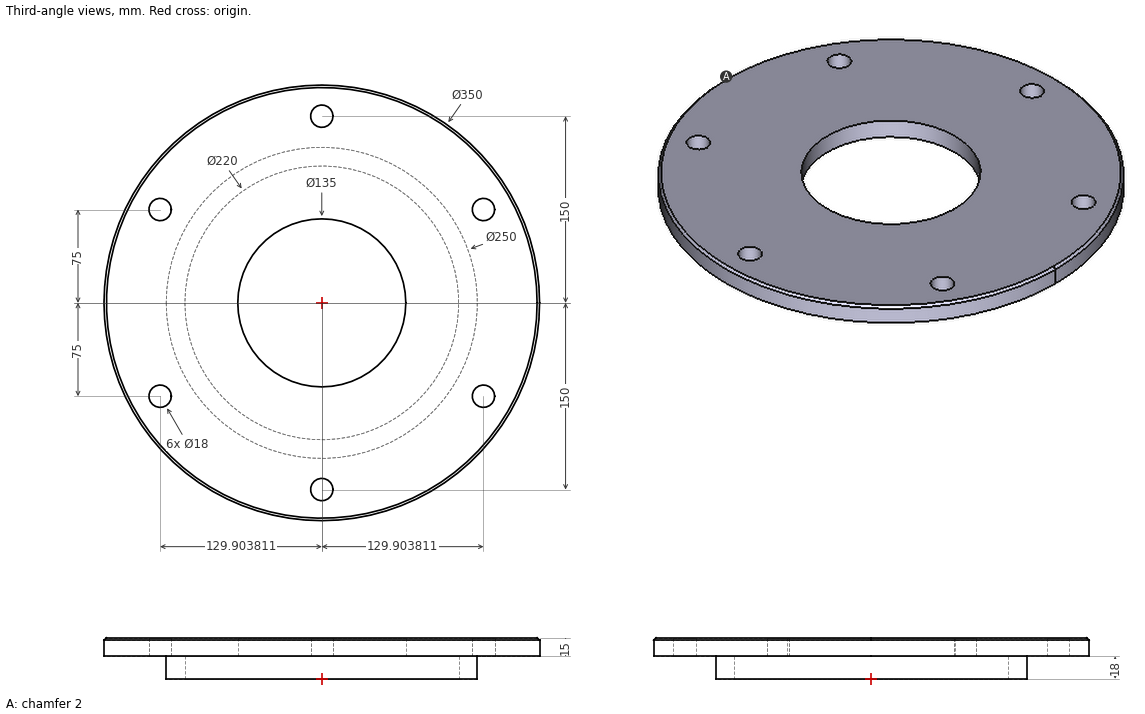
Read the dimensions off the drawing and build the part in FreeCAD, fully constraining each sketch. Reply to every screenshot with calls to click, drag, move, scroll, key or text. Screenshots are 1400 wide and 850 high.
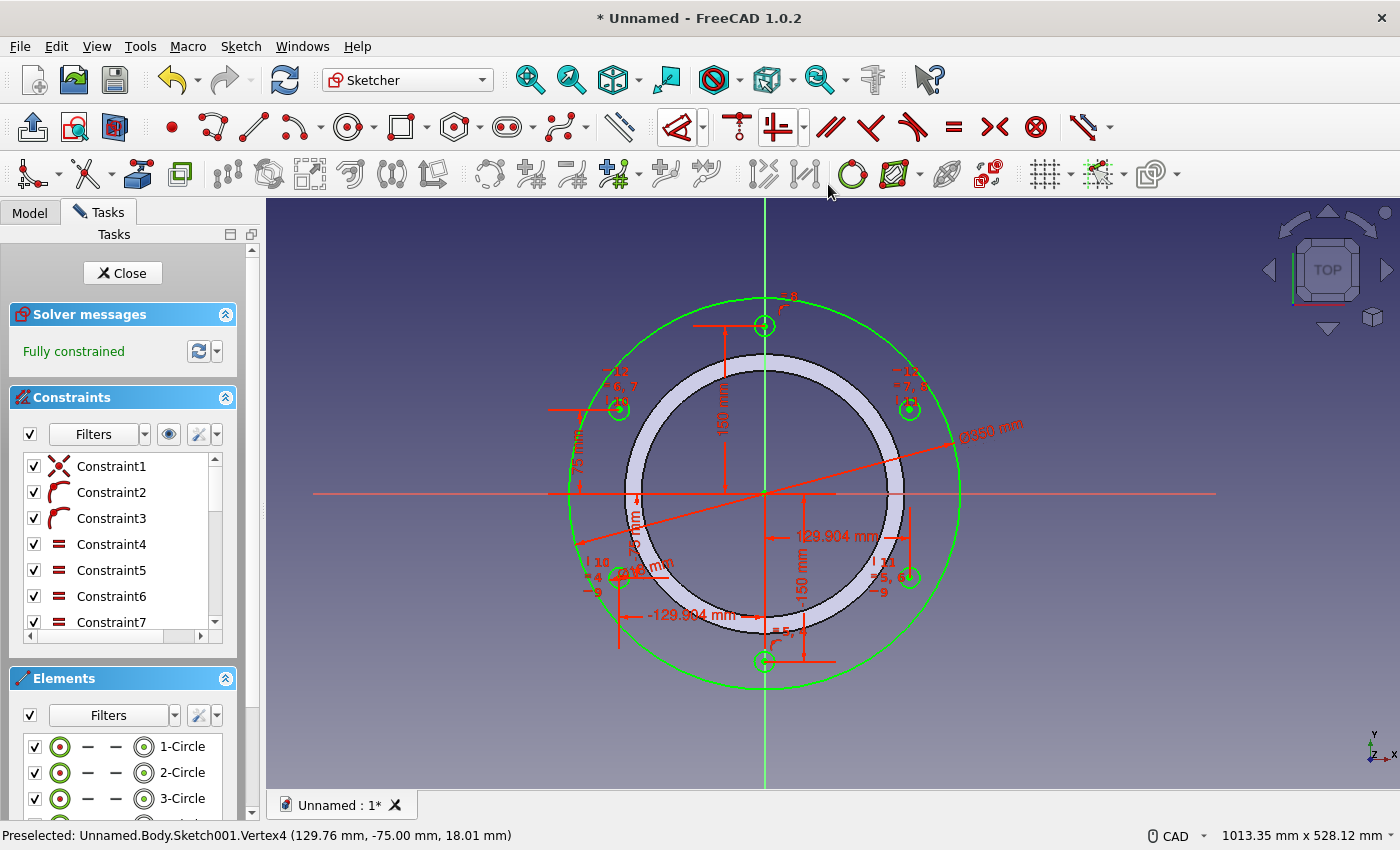
click(123, 273)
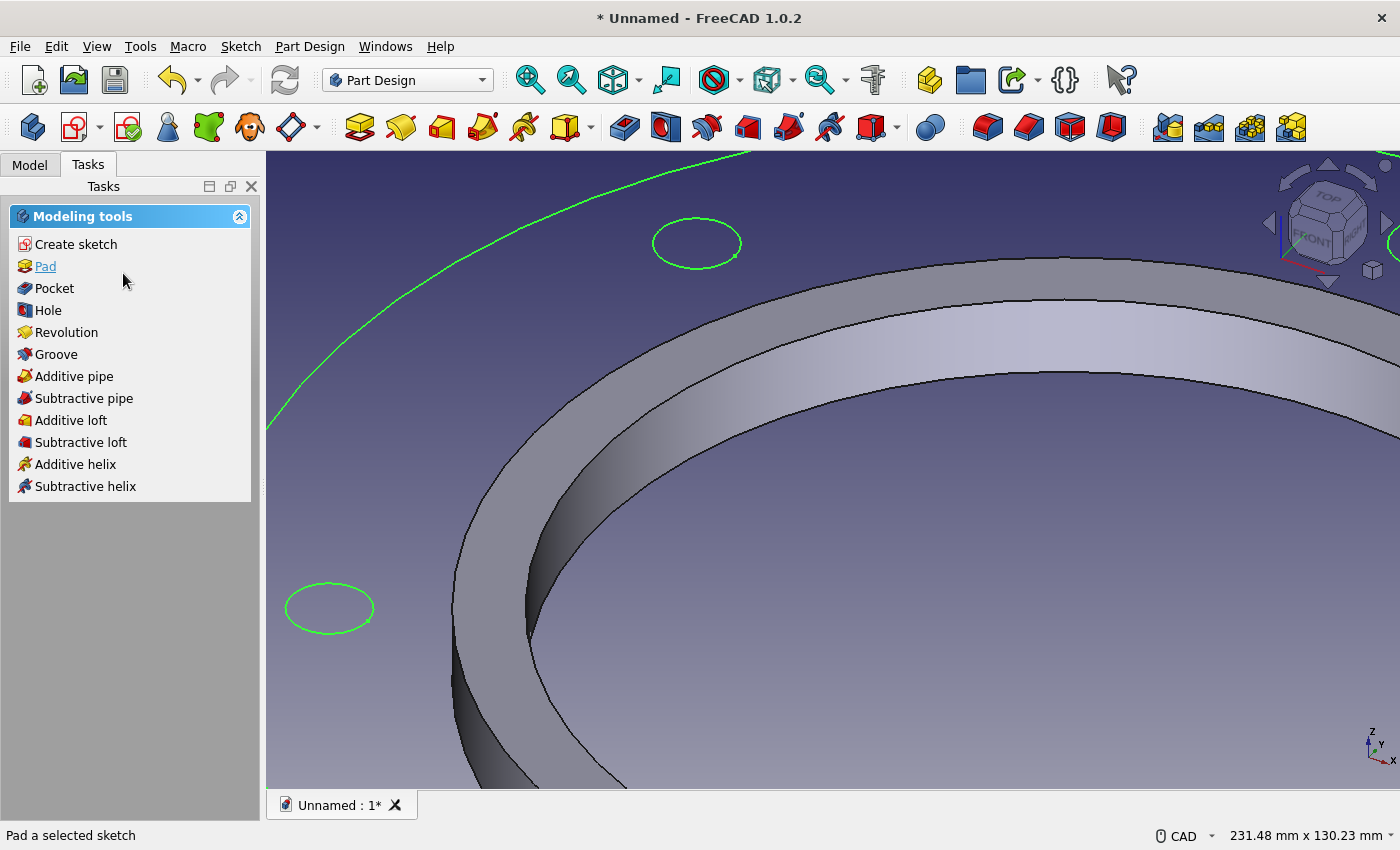
click(360, 128)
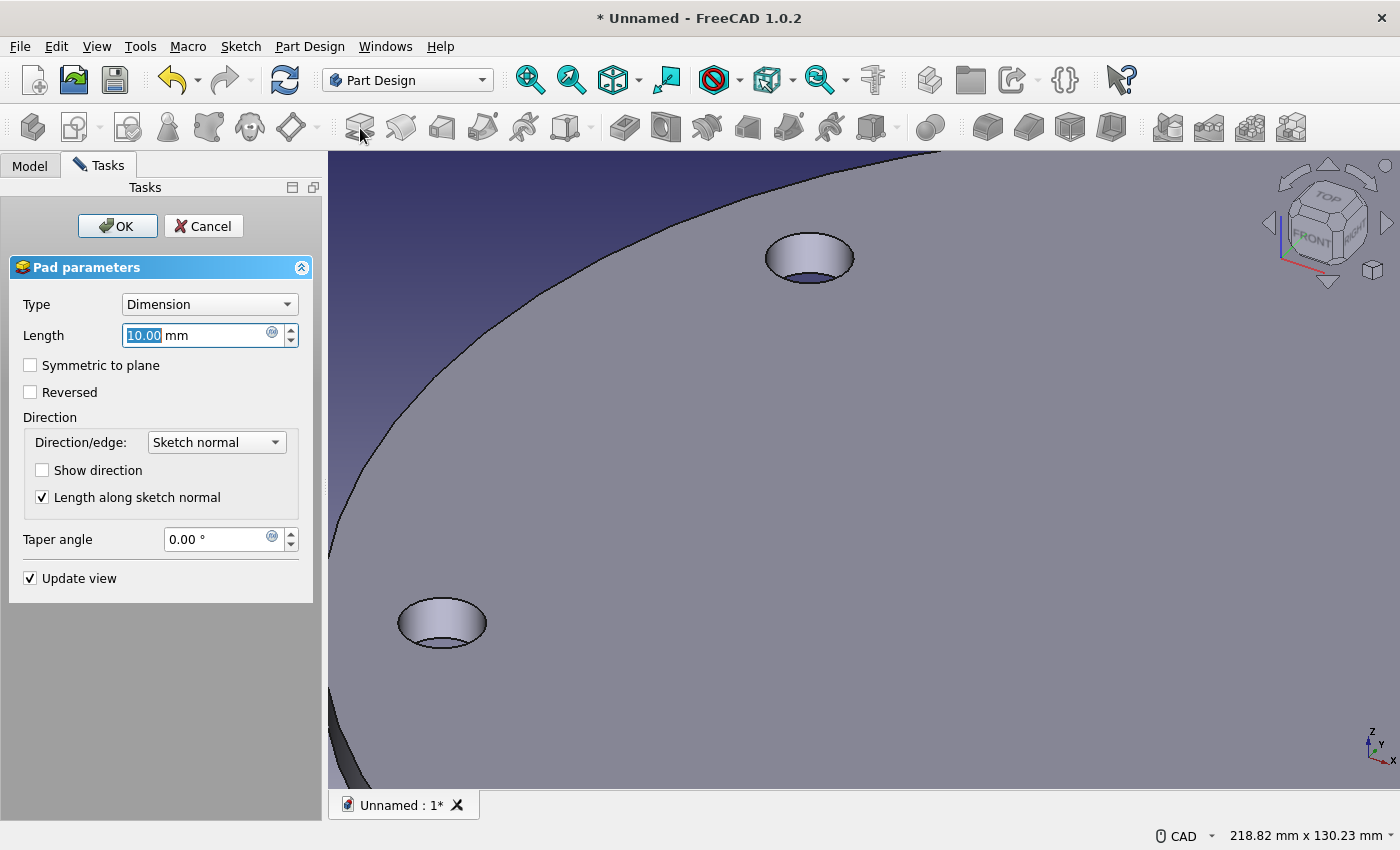
text(15)
key(Tab)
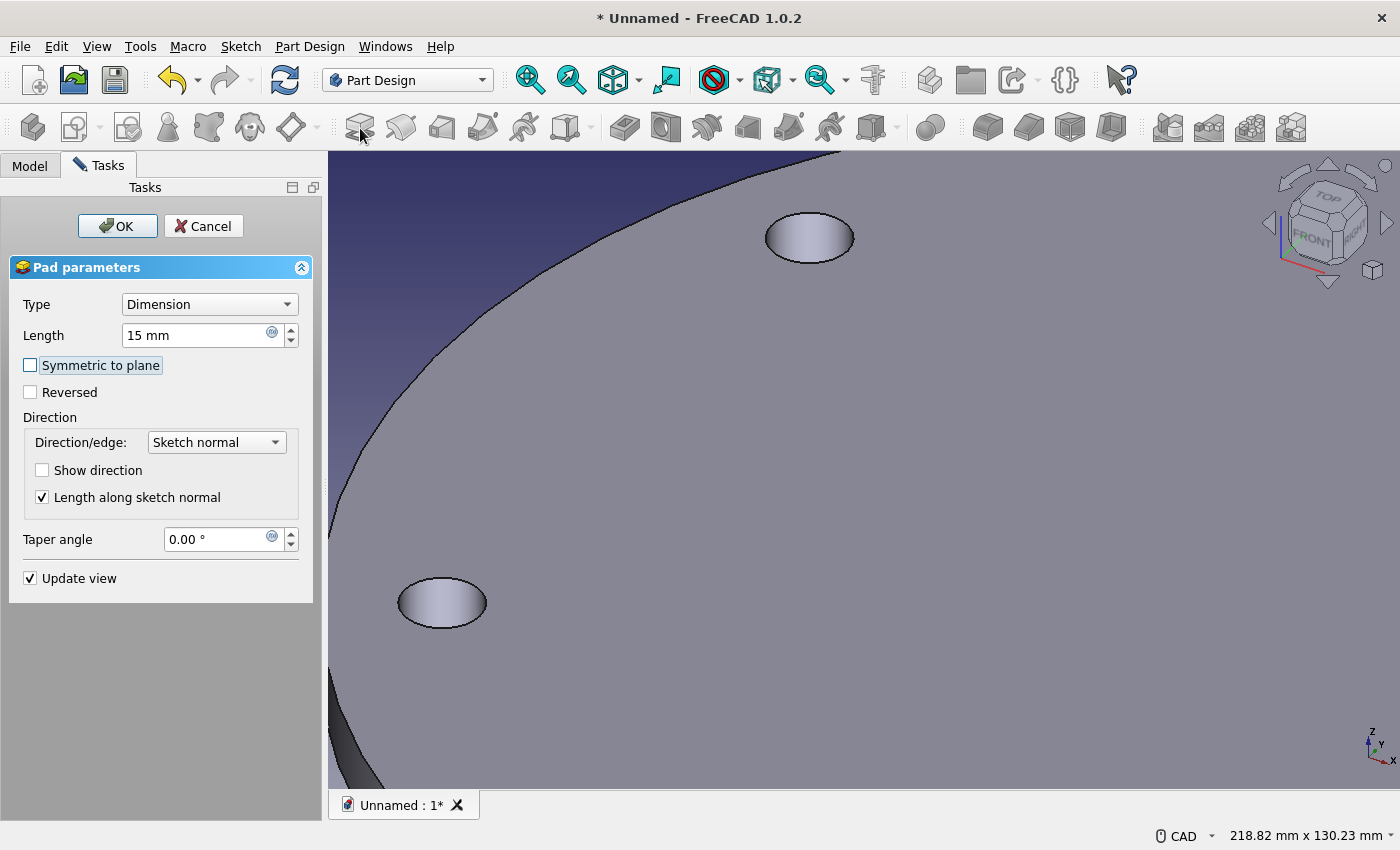
click(118, 226)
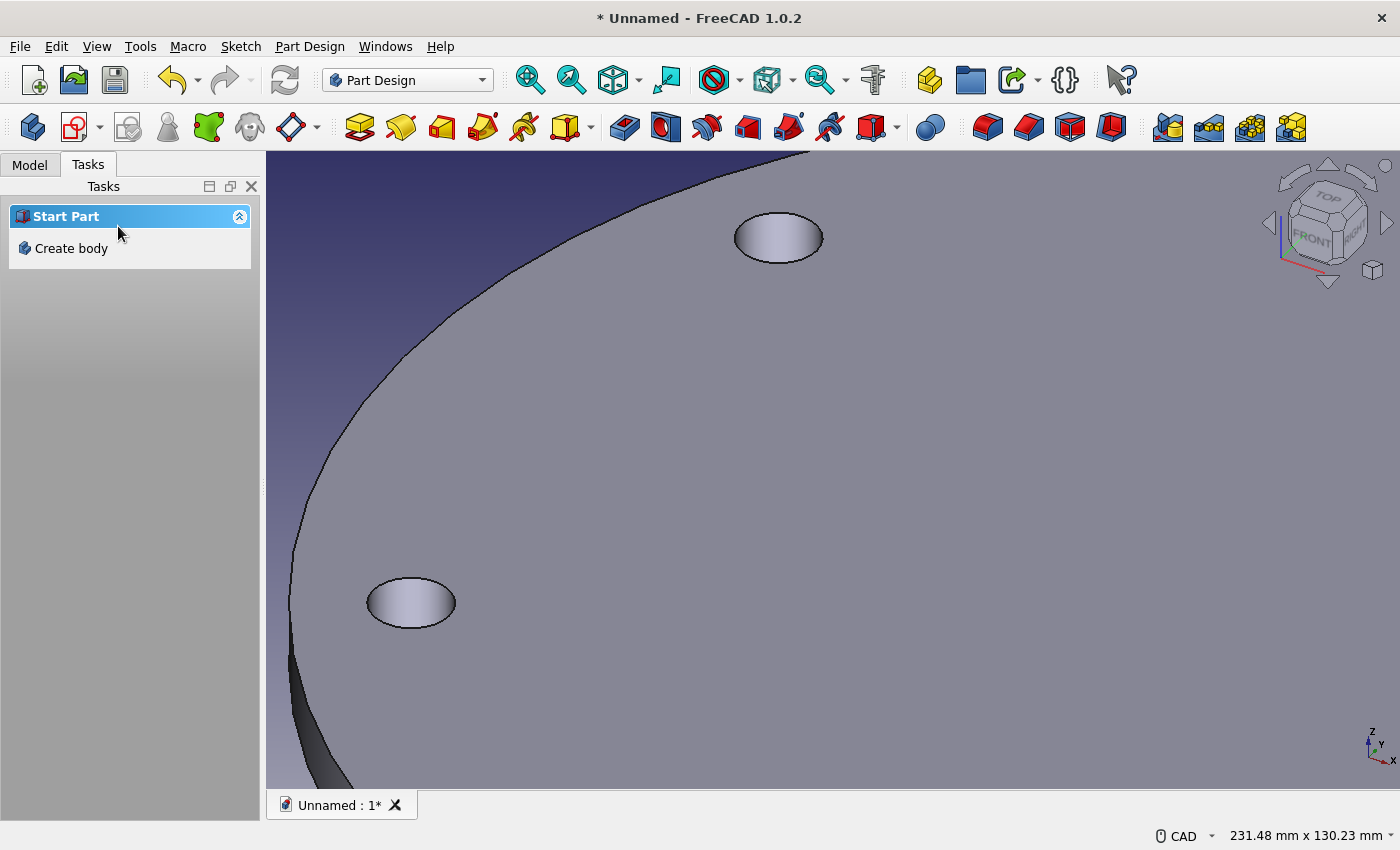
key(v)
key(f)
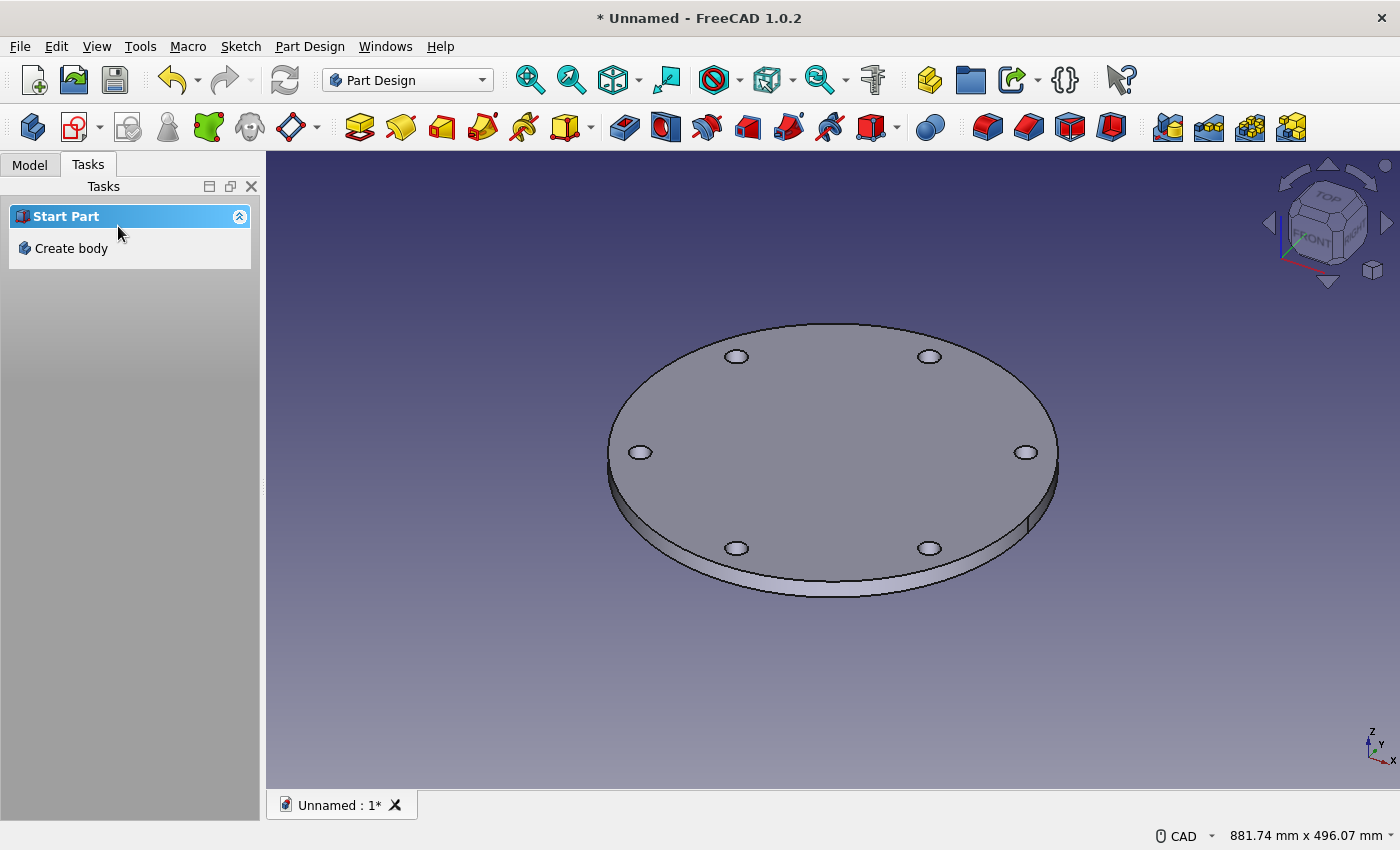
click(609, 465)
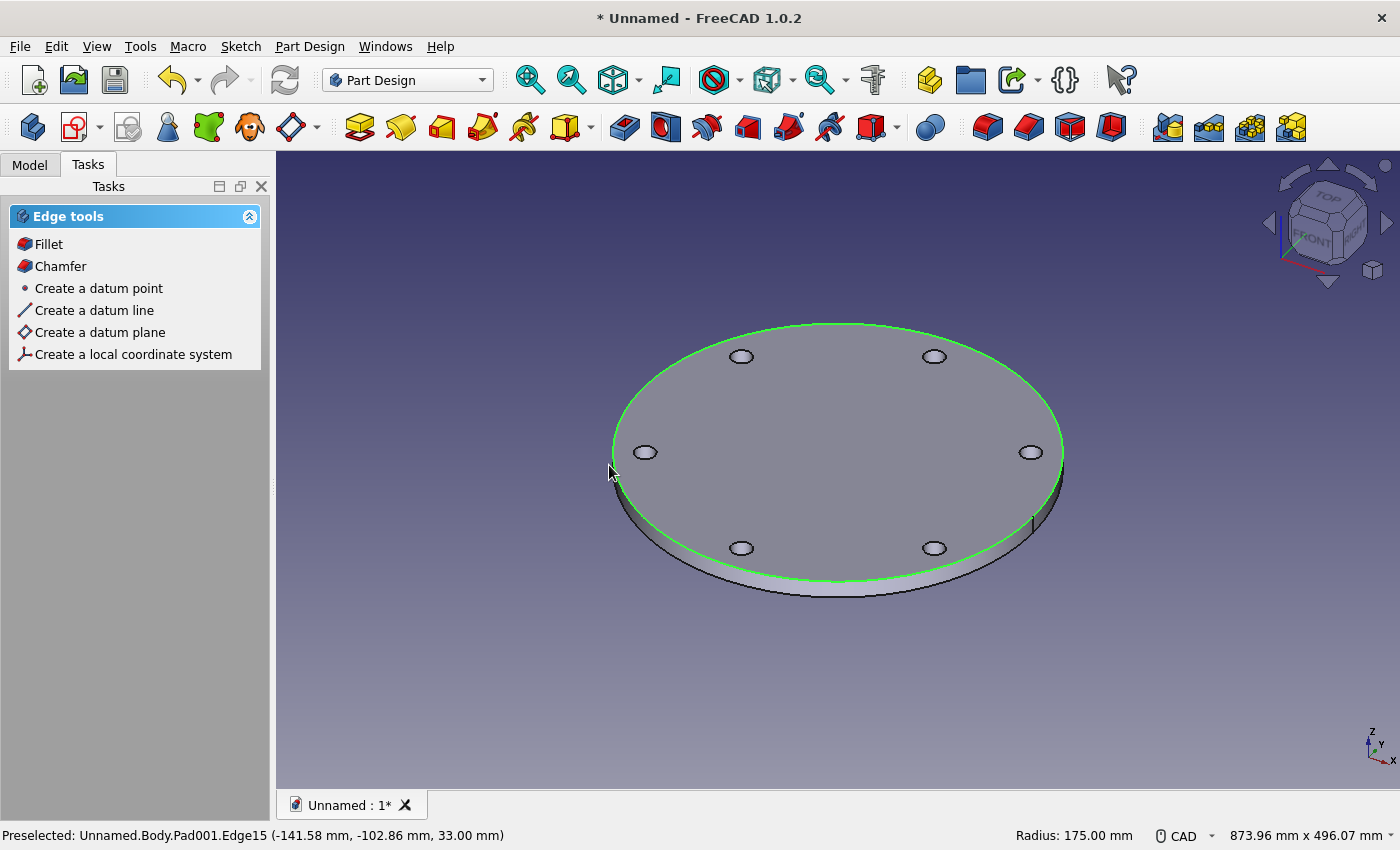
click(1029, 128)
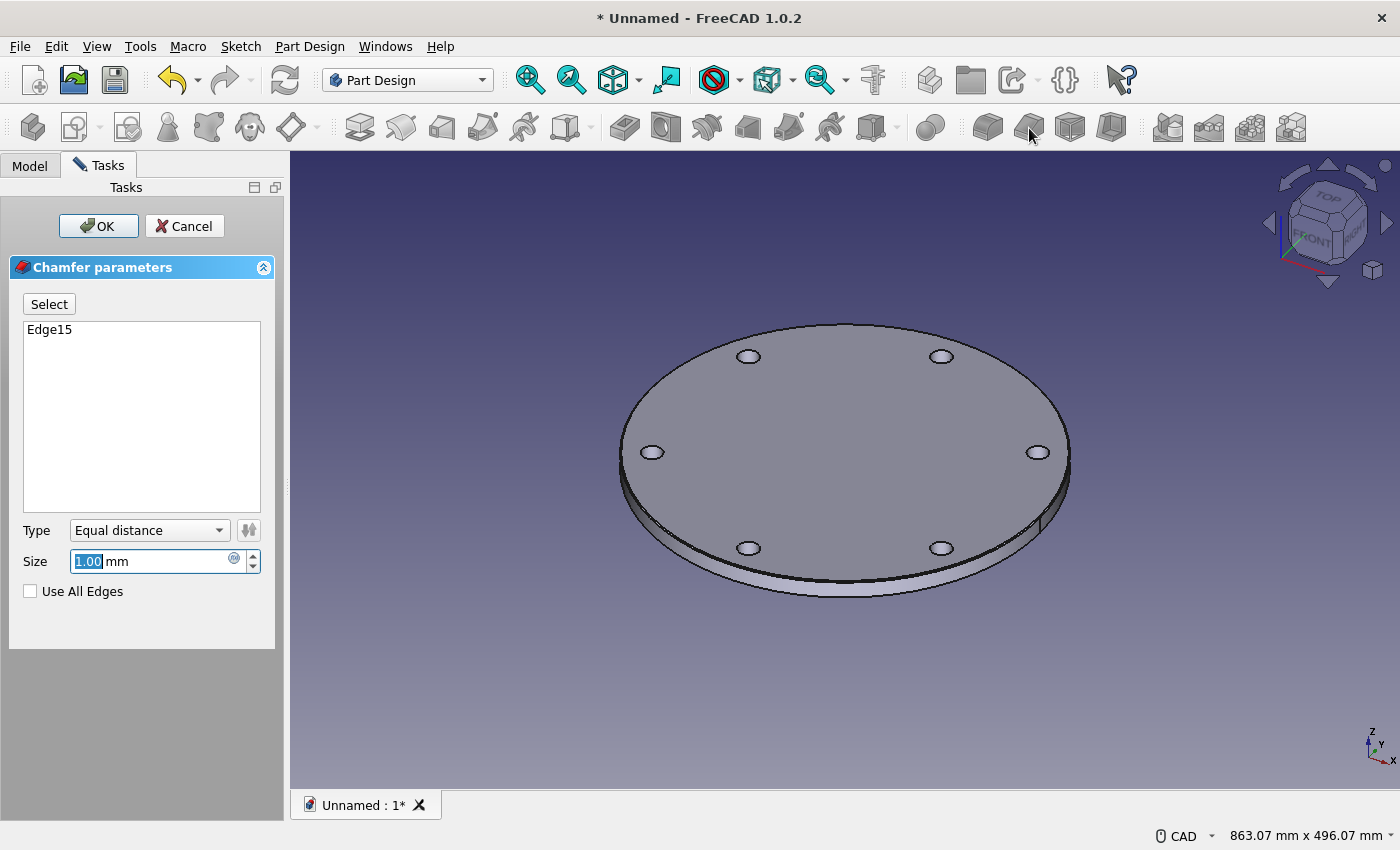
text(2)
key(Tab)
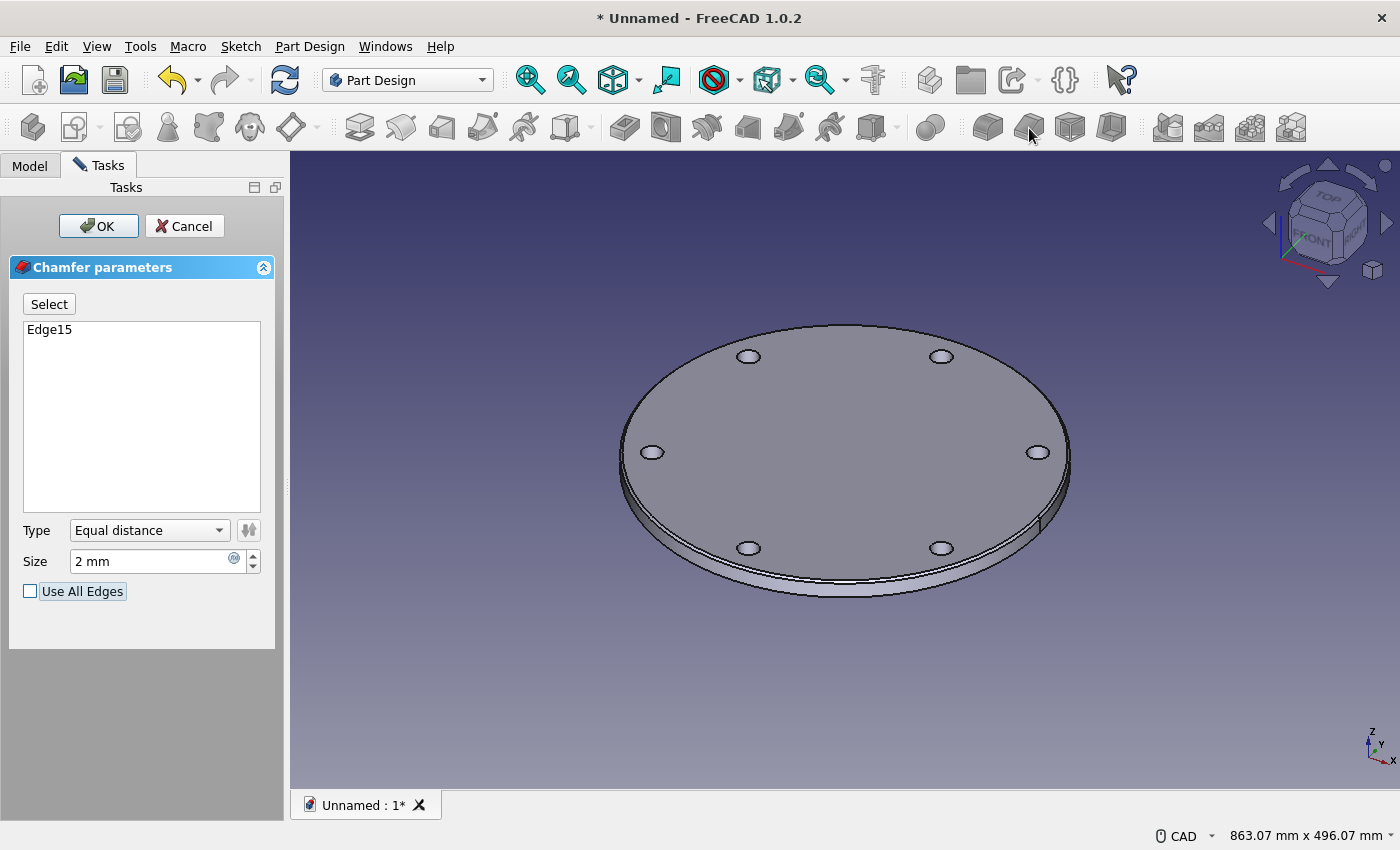
click(99, 226)